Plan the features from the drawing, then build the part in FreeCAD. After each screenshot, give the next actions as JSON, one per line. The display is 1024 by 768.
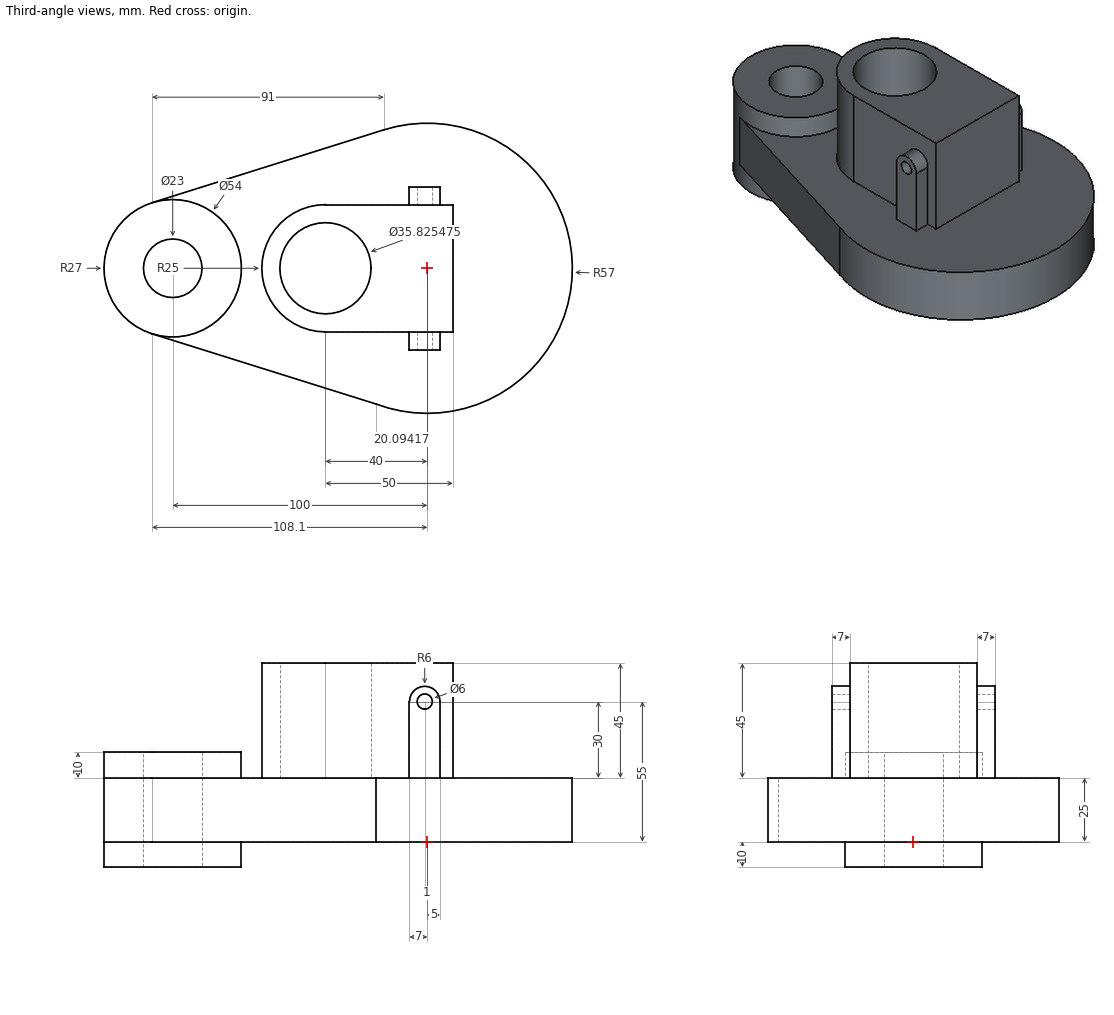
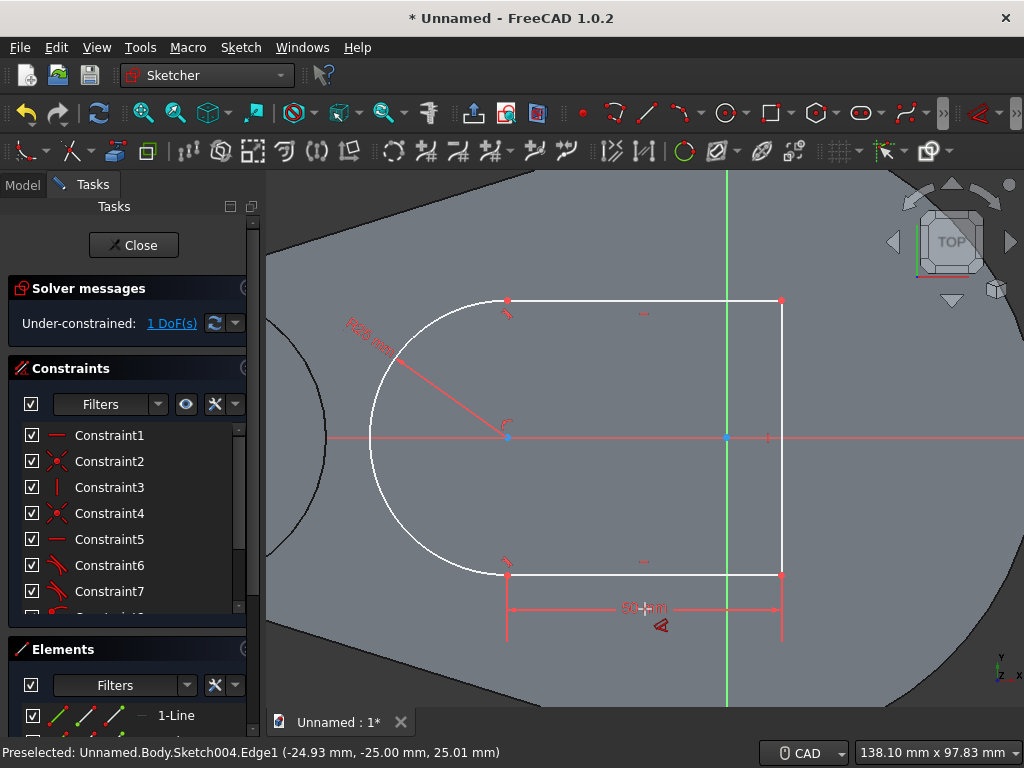
{"action": "left_click", "coordinate": [507, 575]}
{"action": "left_click", "coordinate": [566, 609]}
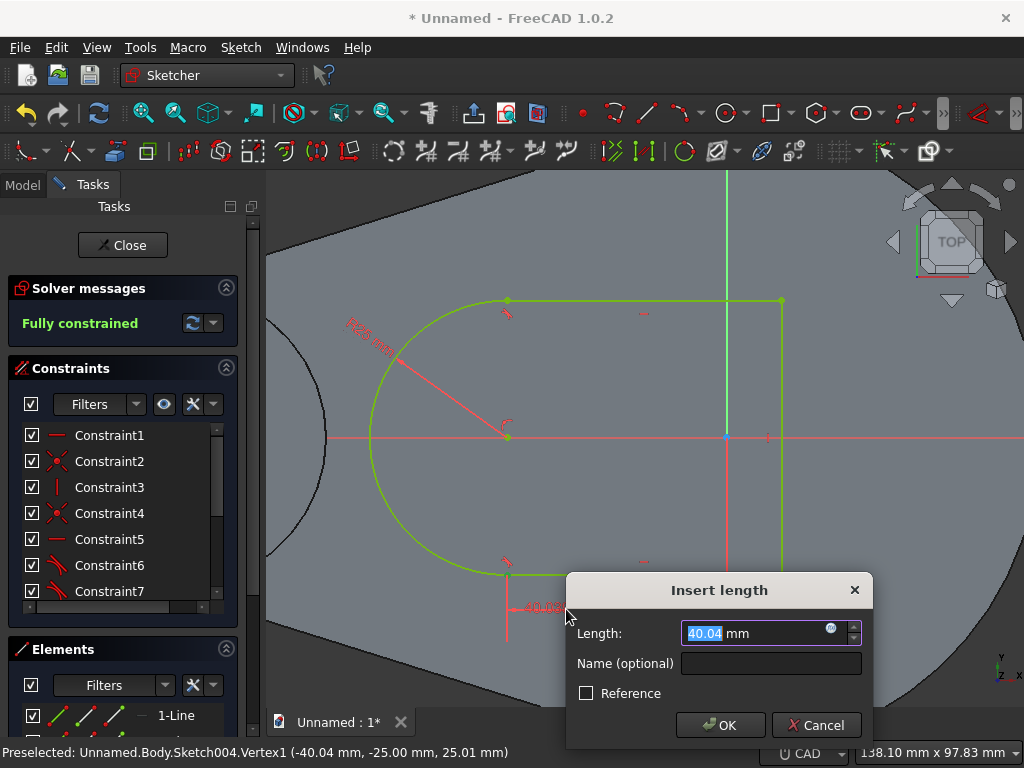
{"action": "type", "text": "40"}
{"action": "key", "text": "Return"}
{"action": "key", "text": "Escape"}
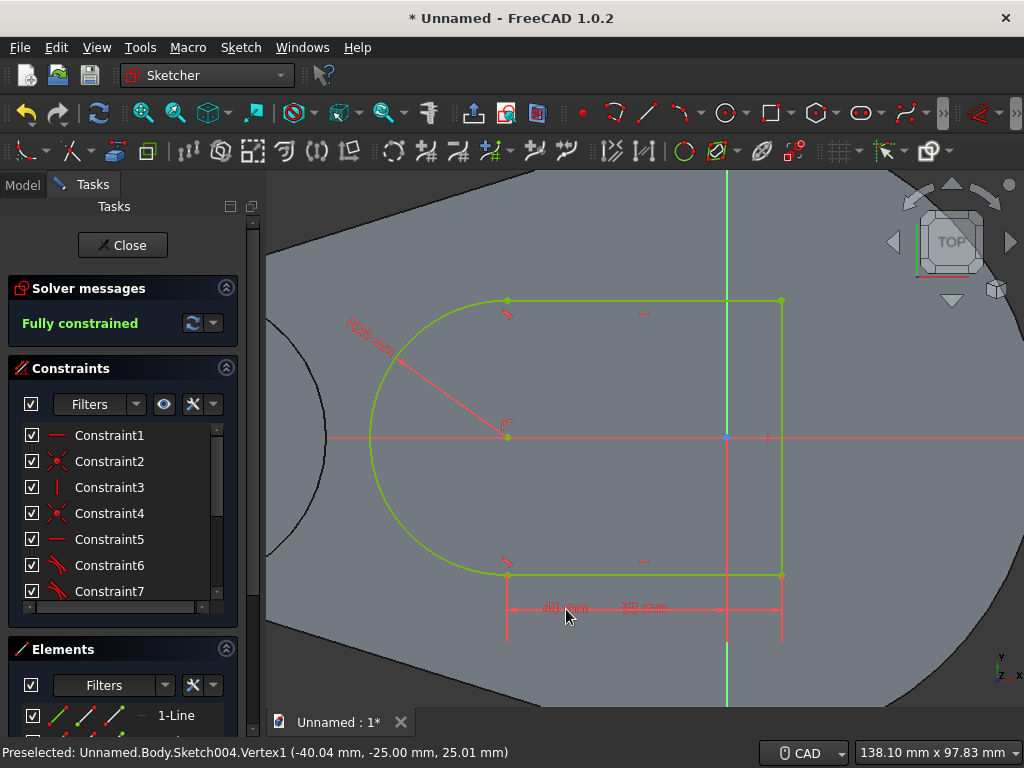
{"action": "left_click", "coordinate": [123, 245]}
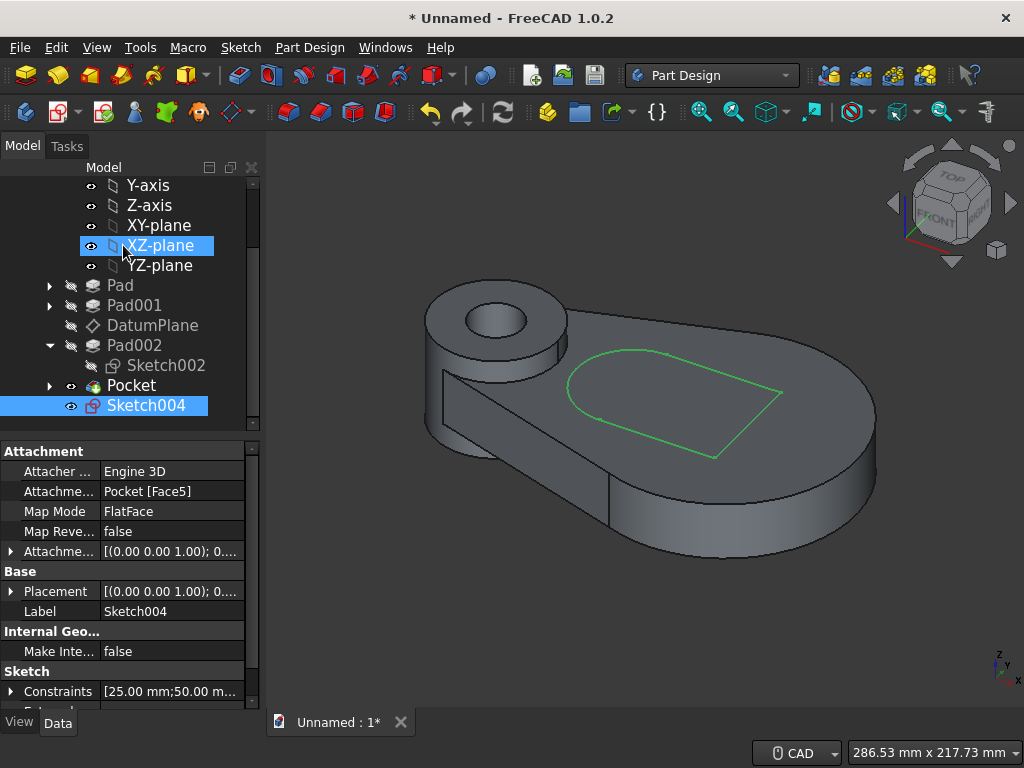
{"action": "left_click", "coordinate": [26, 76]}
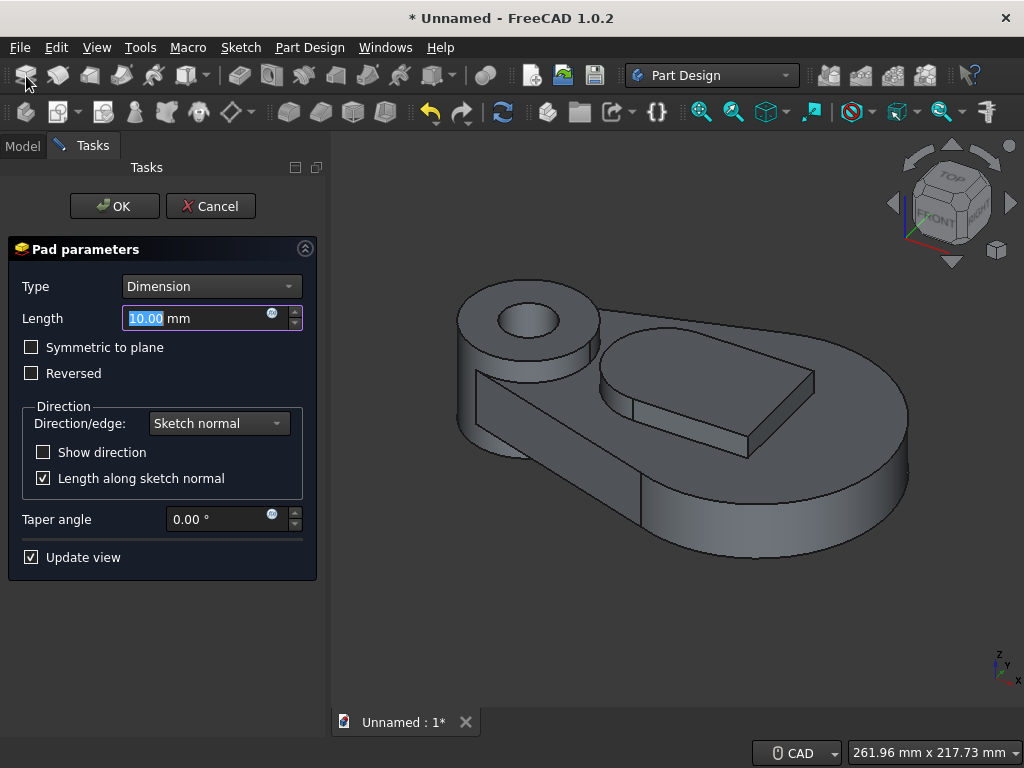
{"action": "type", "text": "45"}
{"action": "key", "text": "Tab"}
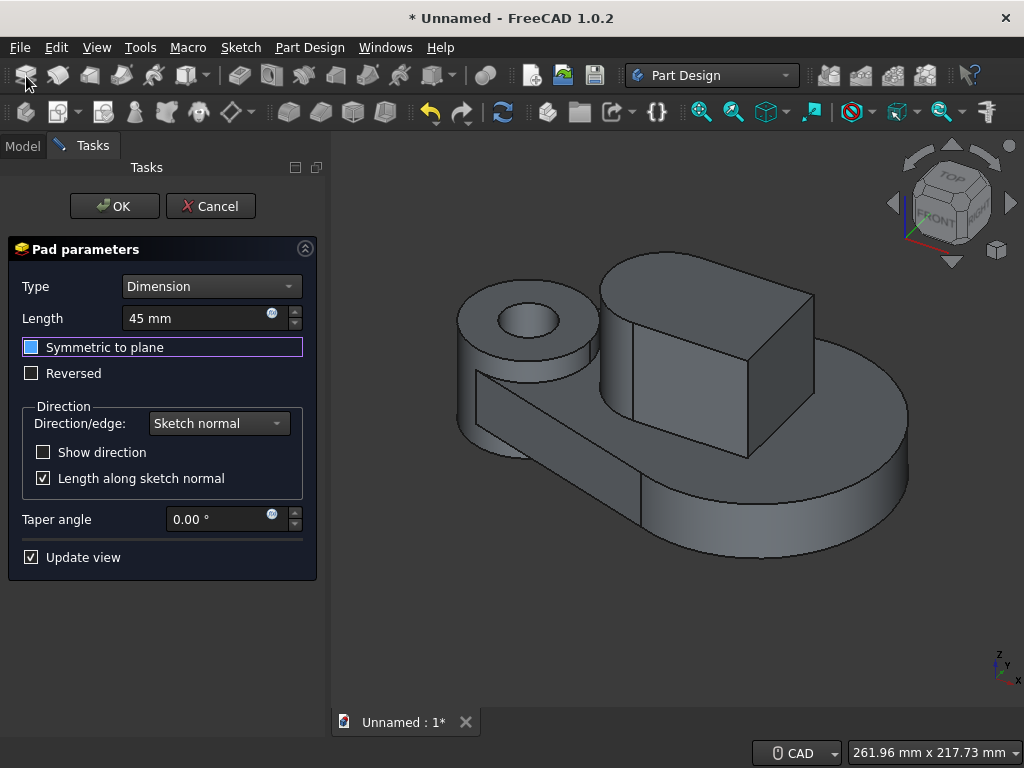
{"action": "left_click", "coordinate": [115, 206]}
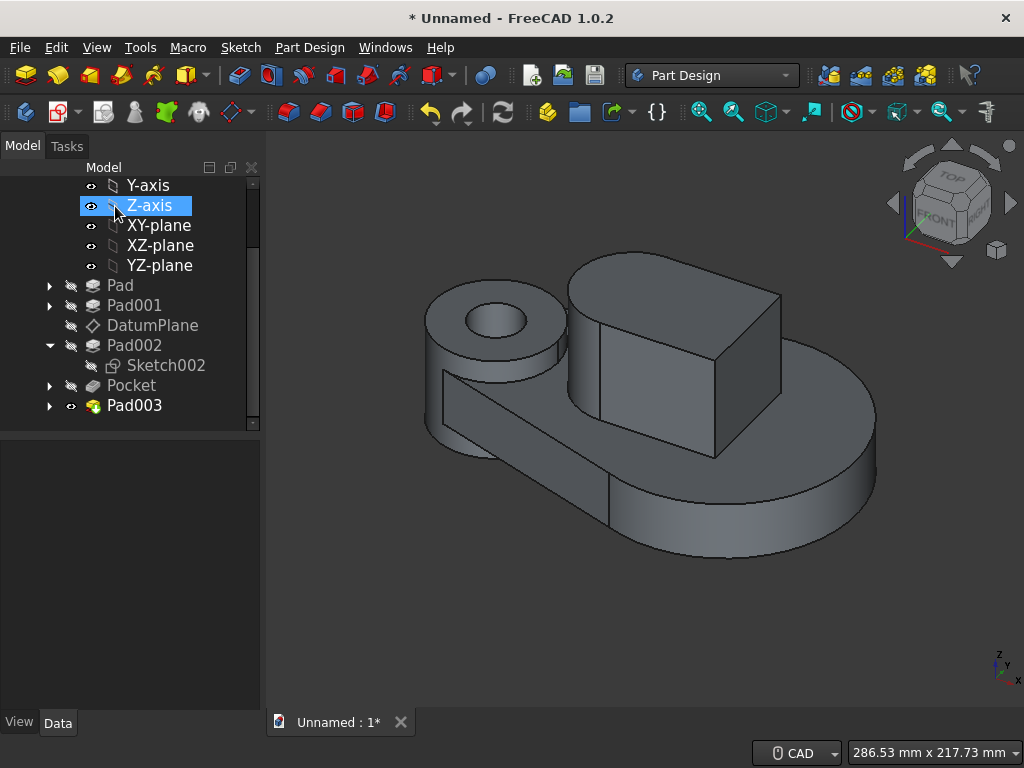
{"action": "left_click", "coordinate": [687, 307]}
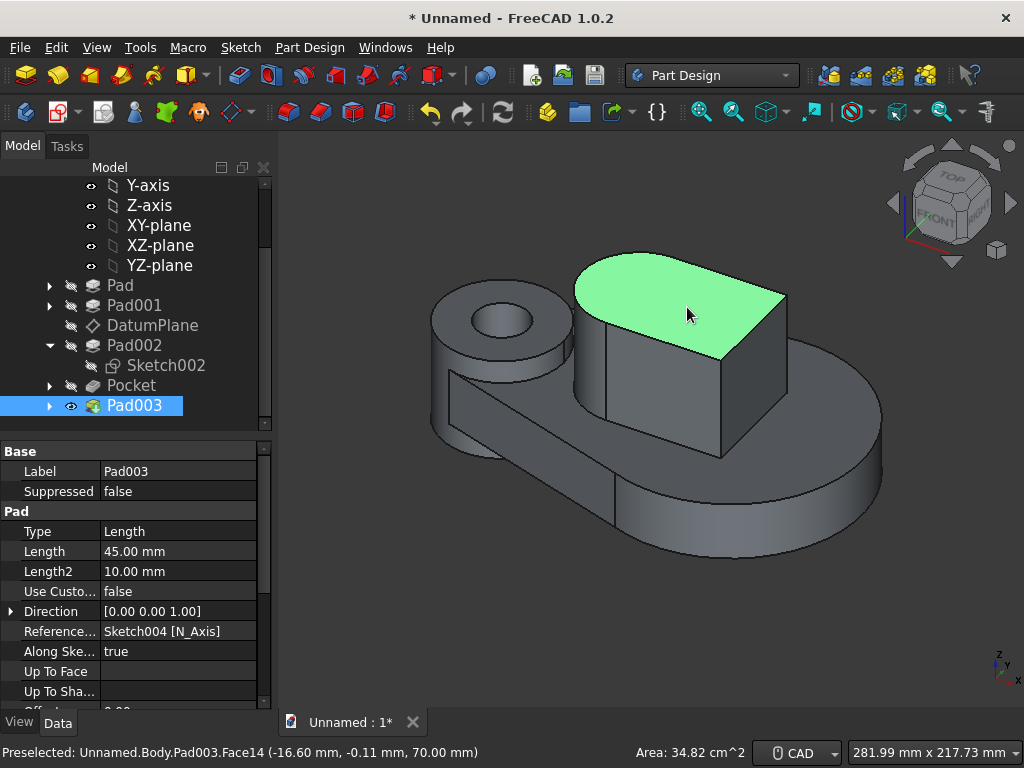
{"action": "left_click", "coordinate": [58, 112]}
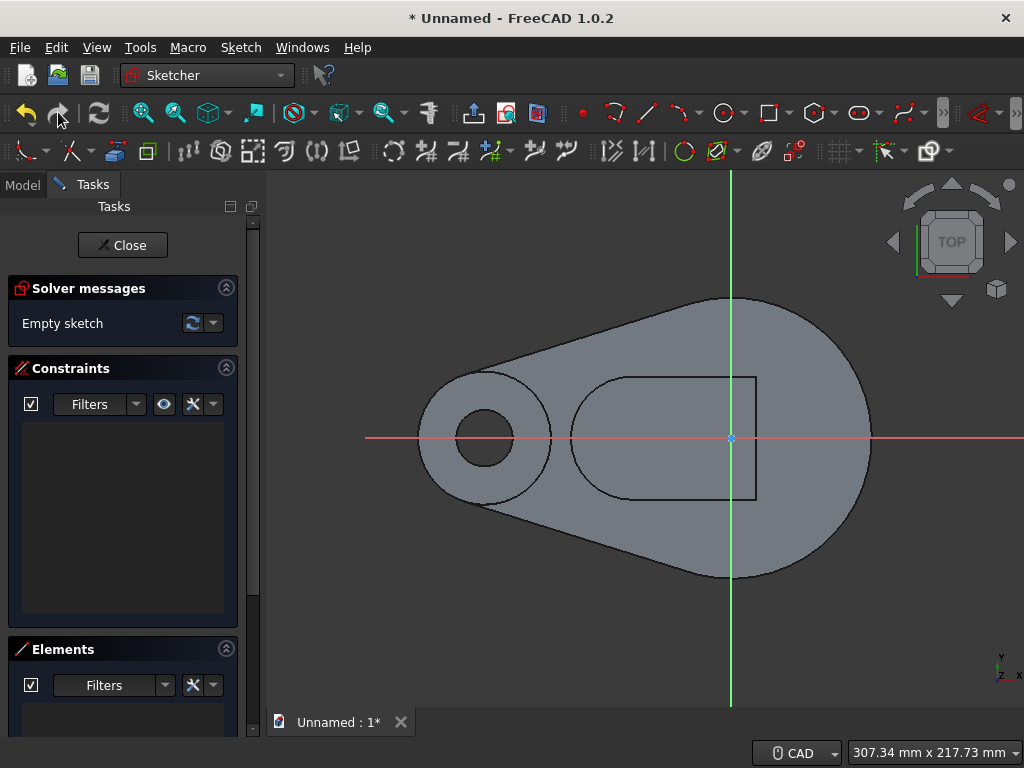
{"action": "scroll", "coordinate": [708, 438], "scroll_direction": "up", "scroll_amount": 5}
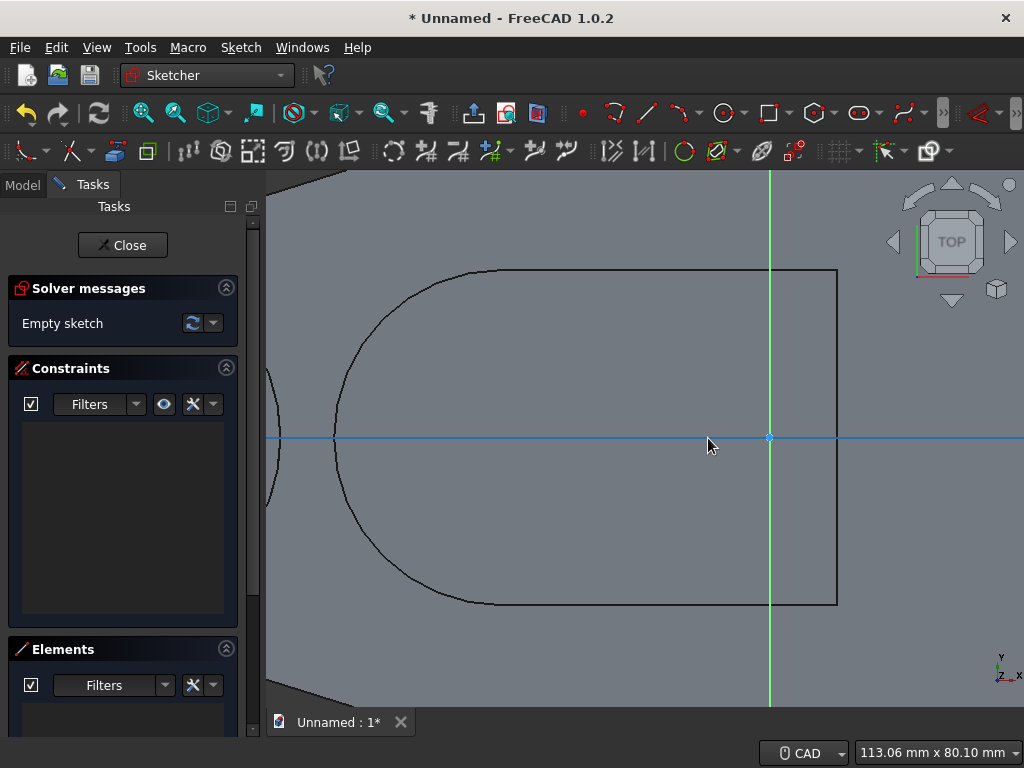
{"action": "key", "text": "g c"}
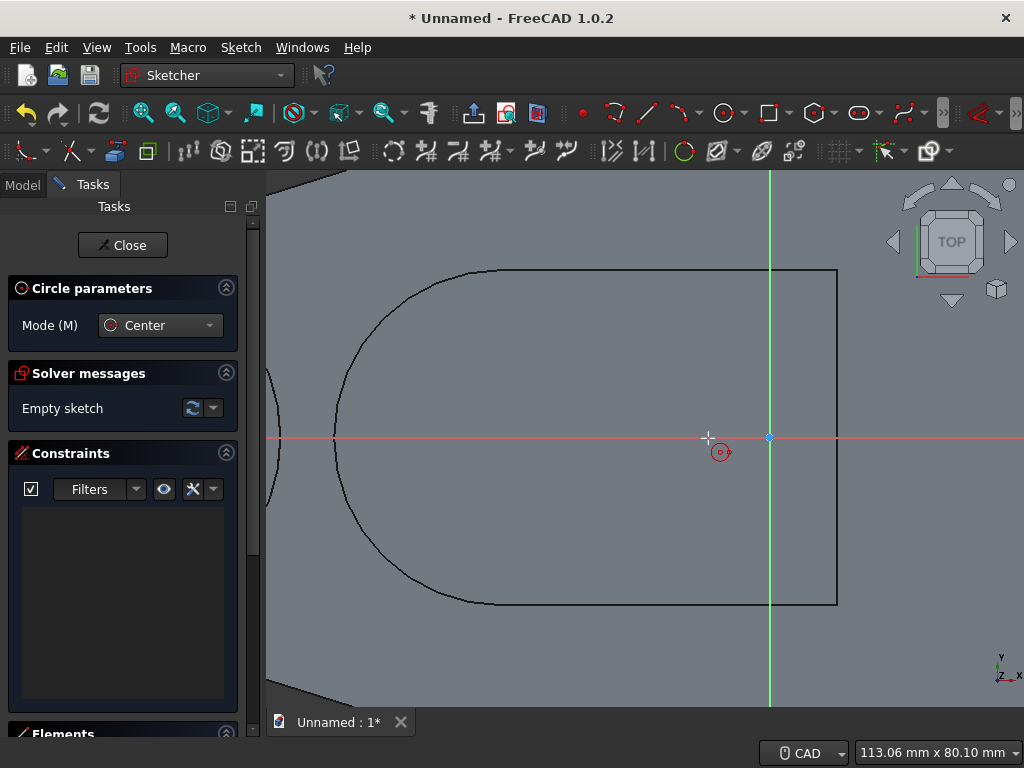
{"action": "left_click", "coordinate": [502, 438]}
{"action": "left_click", "coordinate": [587, 353]}
{"action": "key", "text": "Escape"}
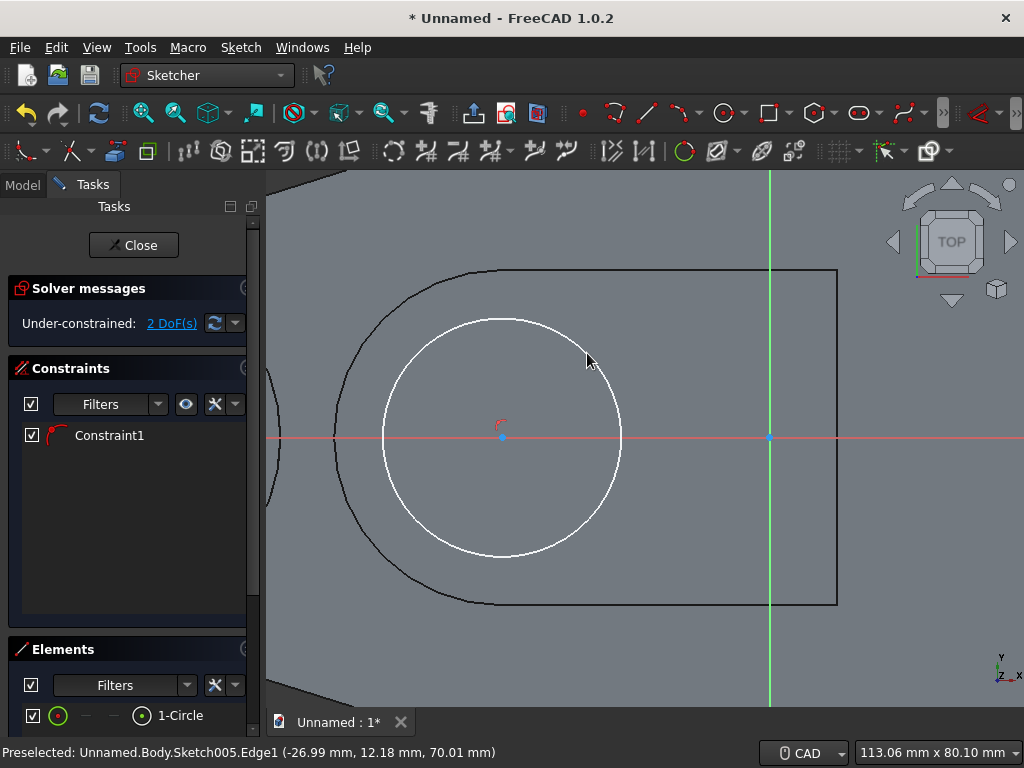
{"action": "key", "text": "d"}